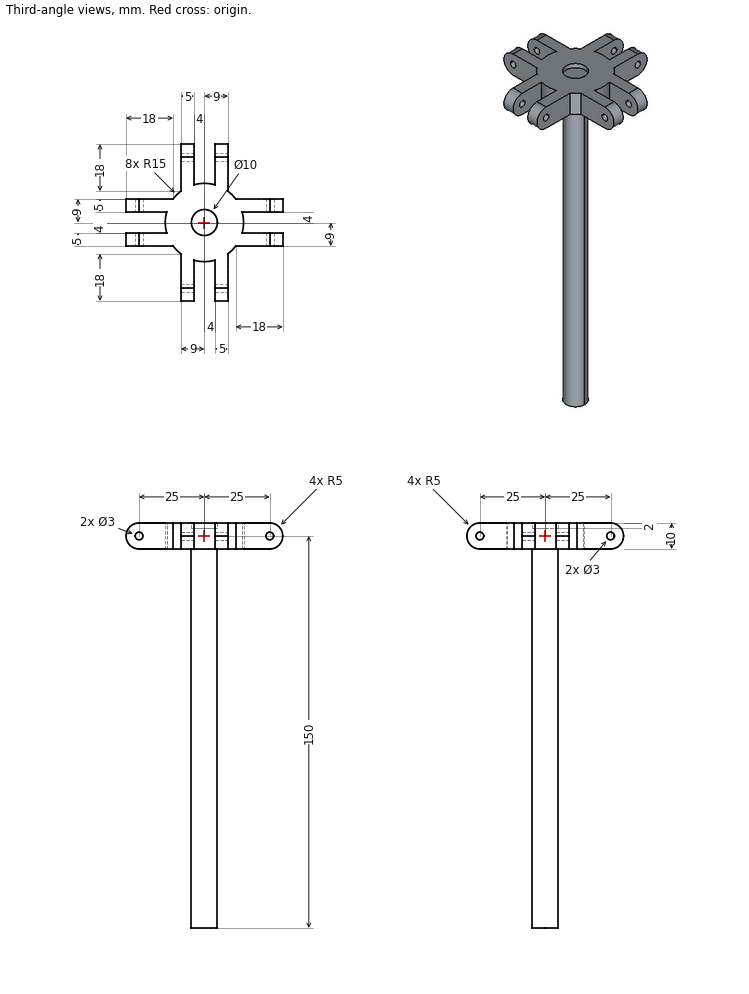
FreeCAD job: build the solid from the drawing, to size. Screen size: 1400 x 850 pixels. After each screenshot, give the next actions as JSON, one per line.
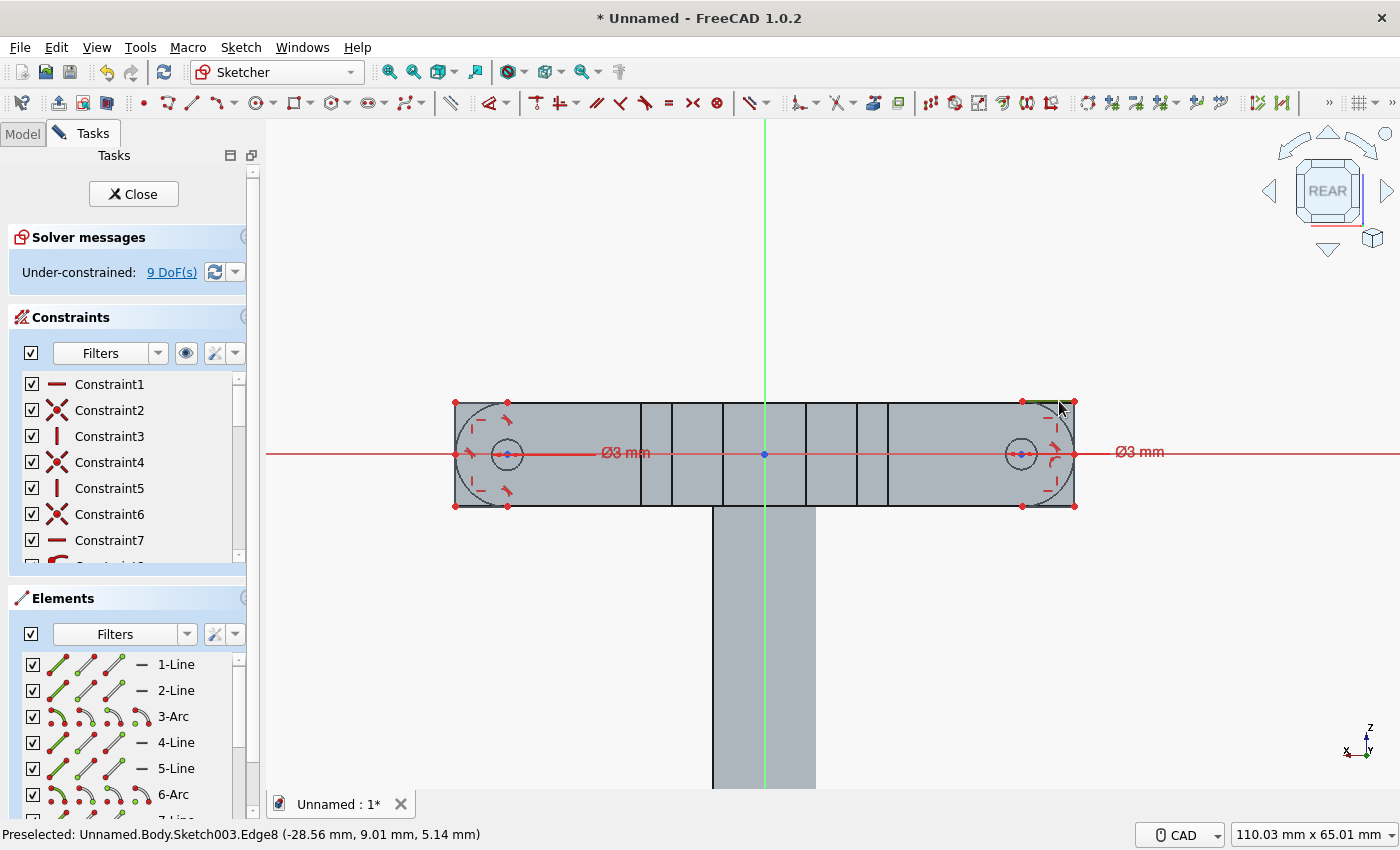
{"action": "left_click", "coordinate": [1059, 417]}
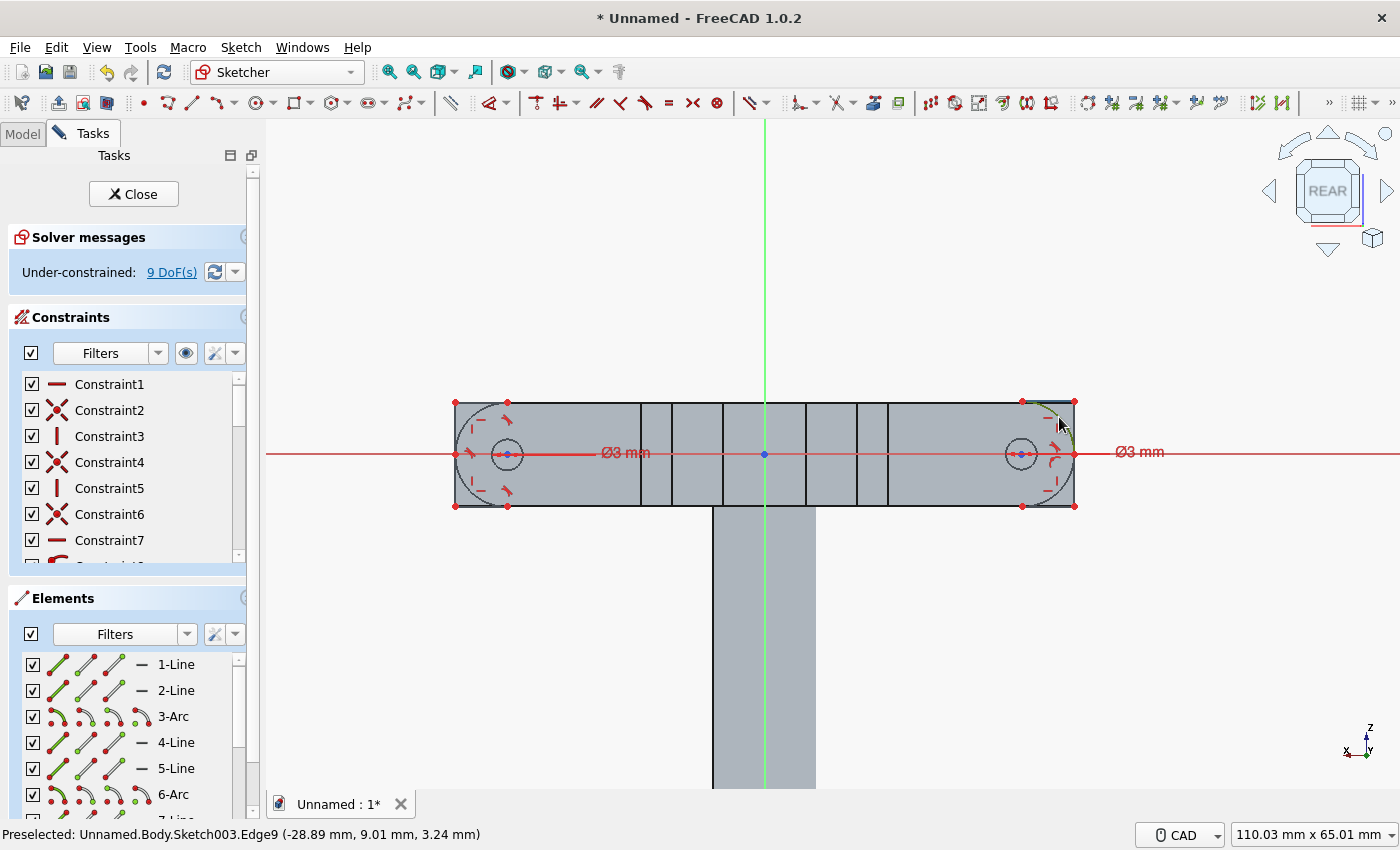
{"action": "key", "text": "t"}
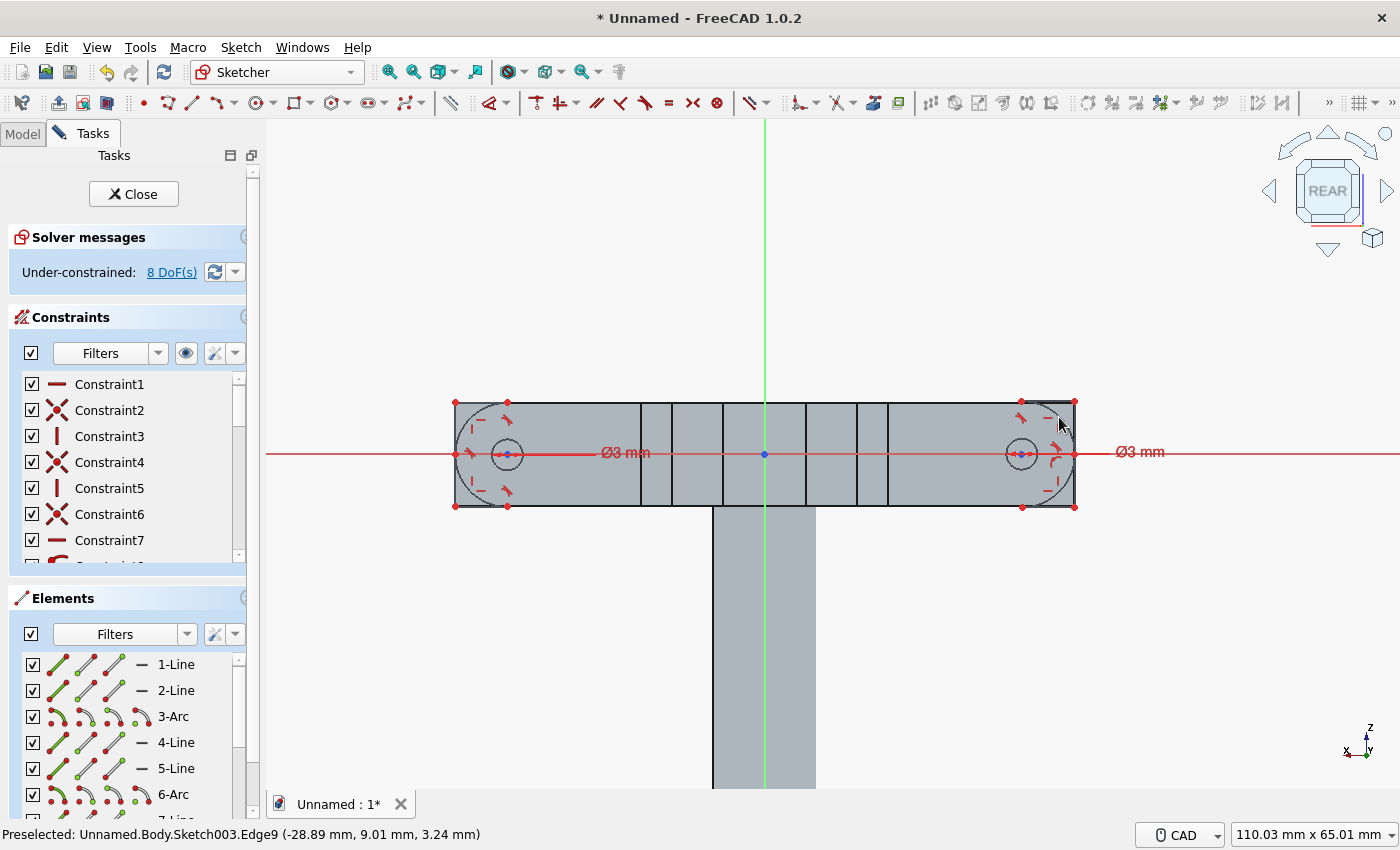
{"action": "left_click", "coordinate": [1059, 507]}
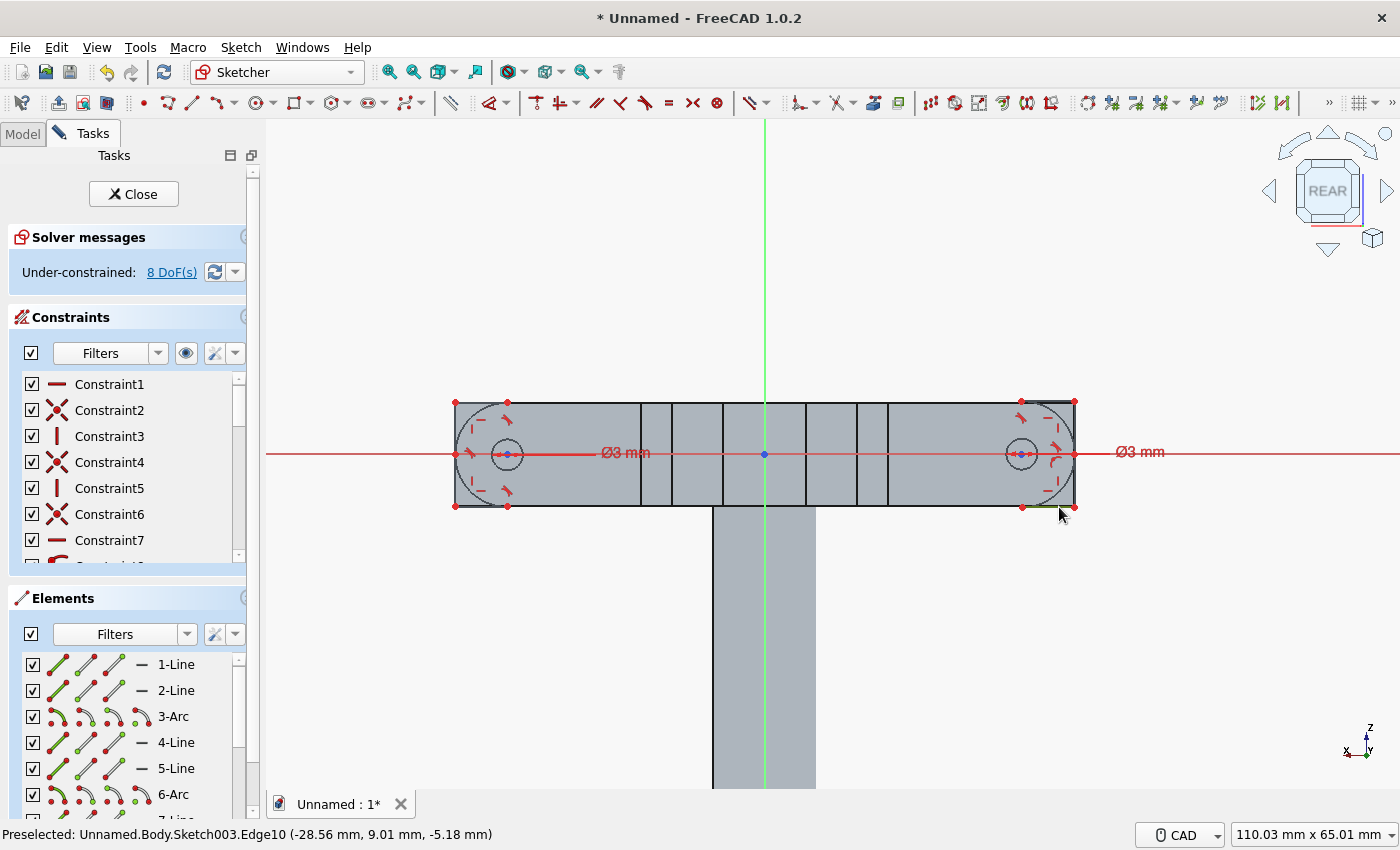
{"action": "left_click", "coordinate": [1059, 492]}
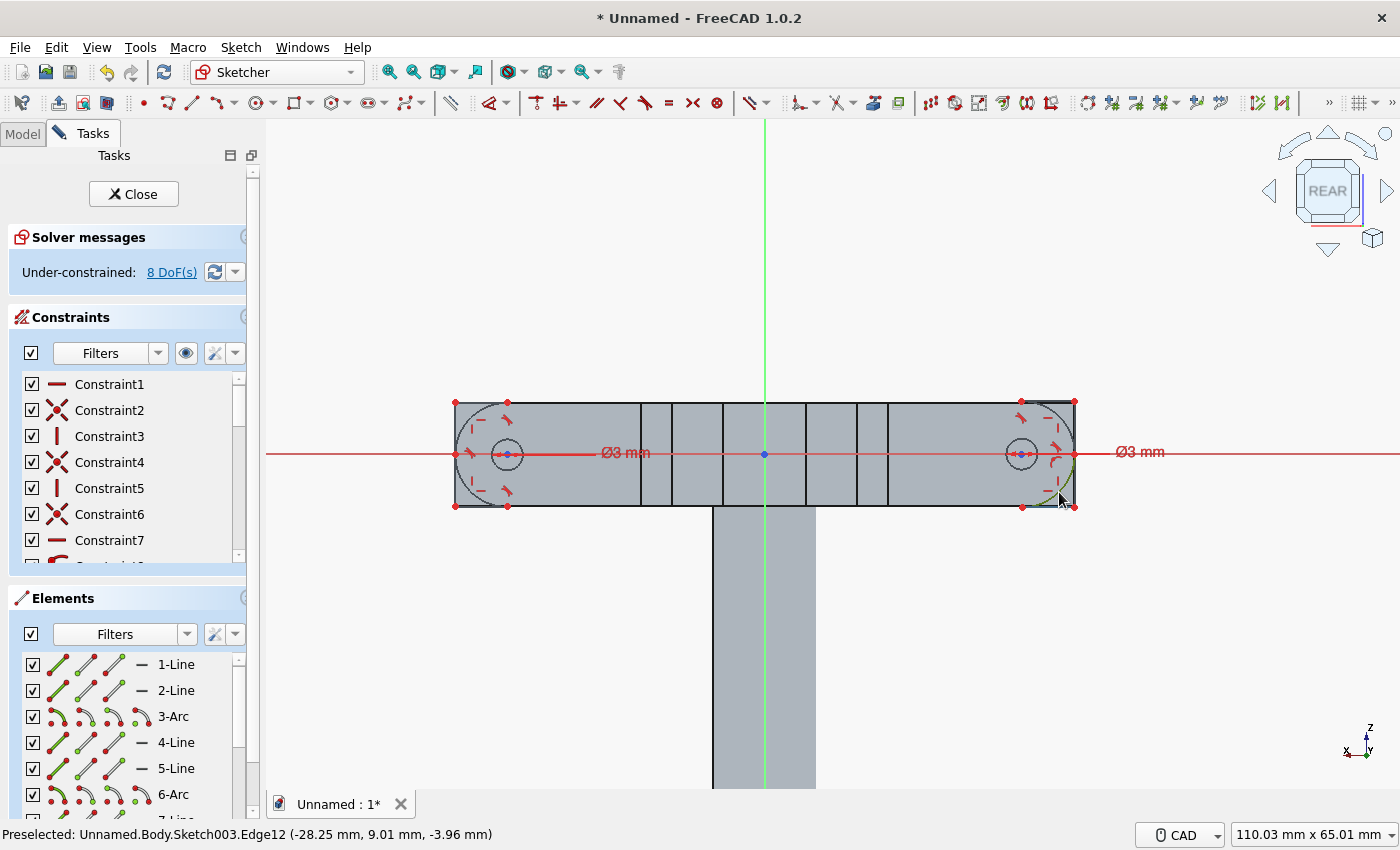
{"action": "key", "text": "t"}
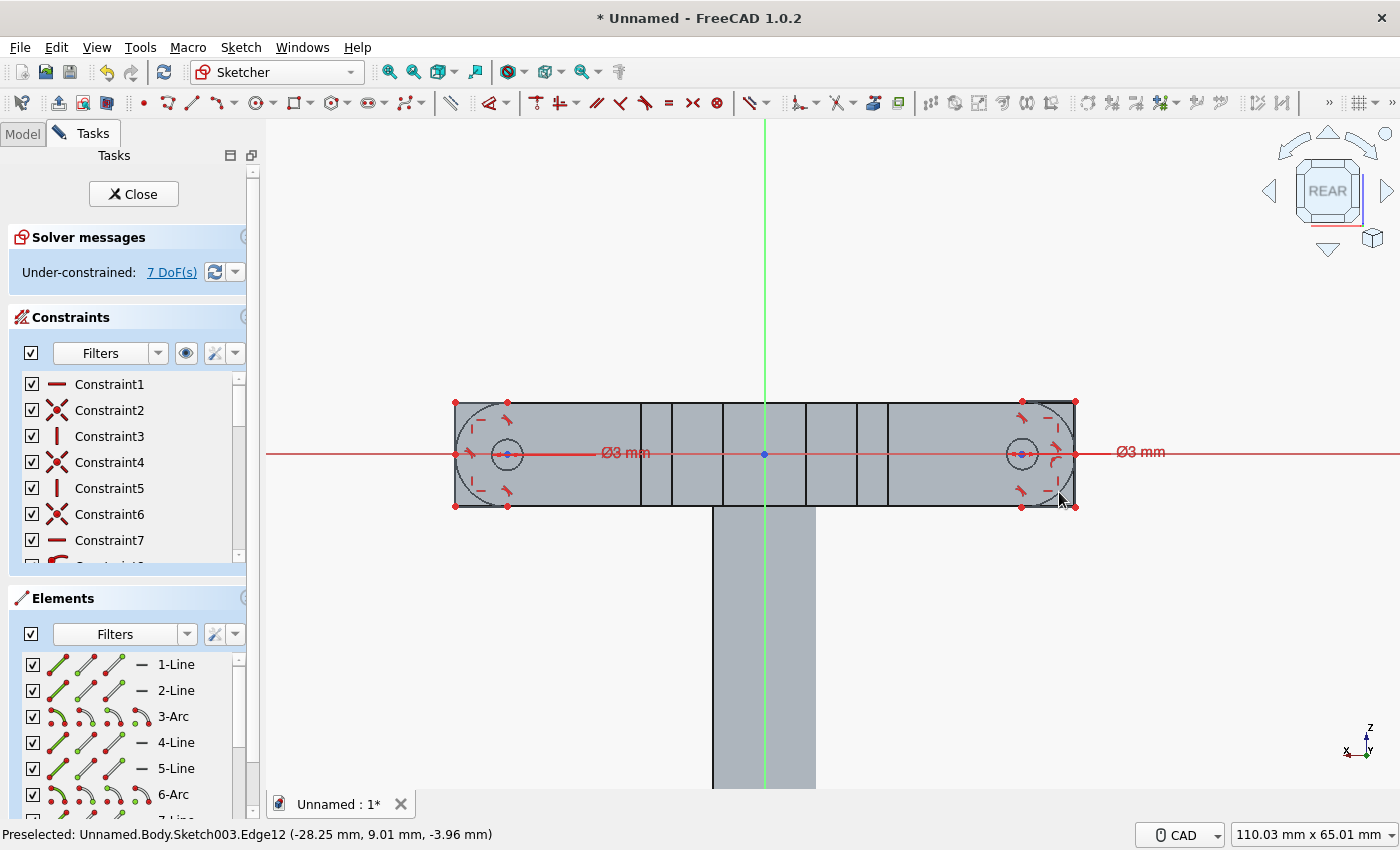
{"action": "left_click", "coordinate": [471, 418]}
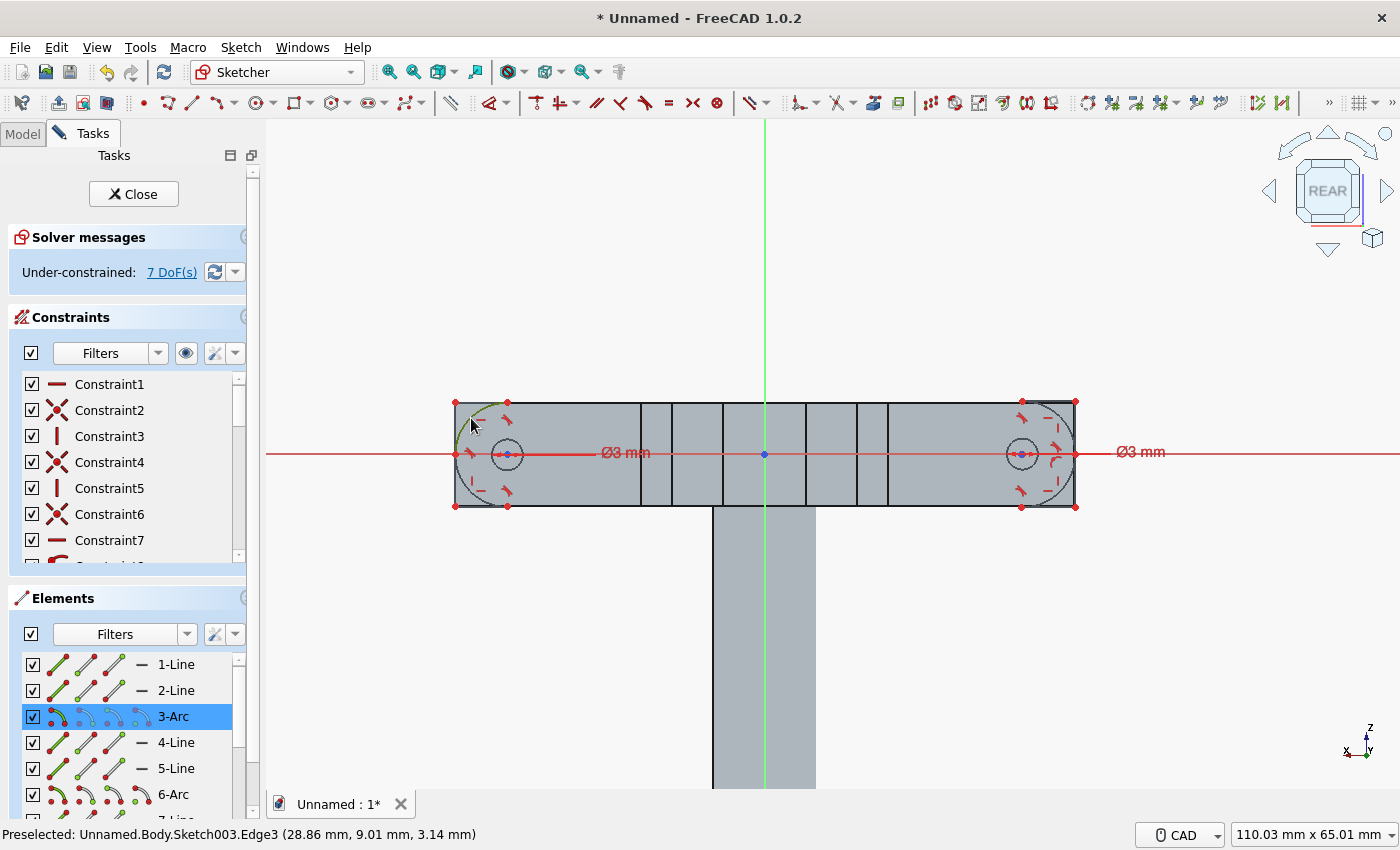
{"action": "left_click", "coordinate": [471, 492]}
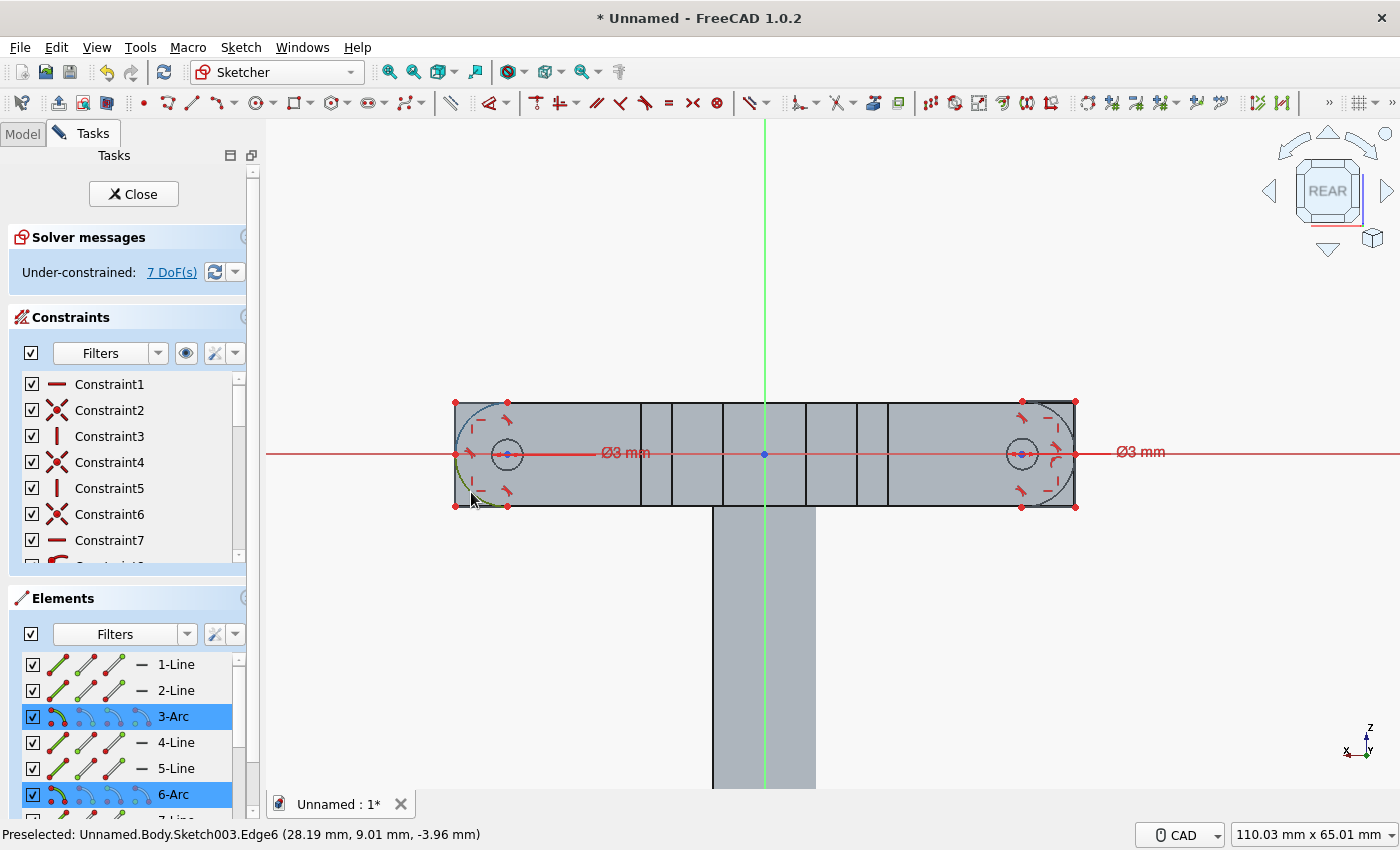
{"action": "left_click", "coordinate": [1060, 417]}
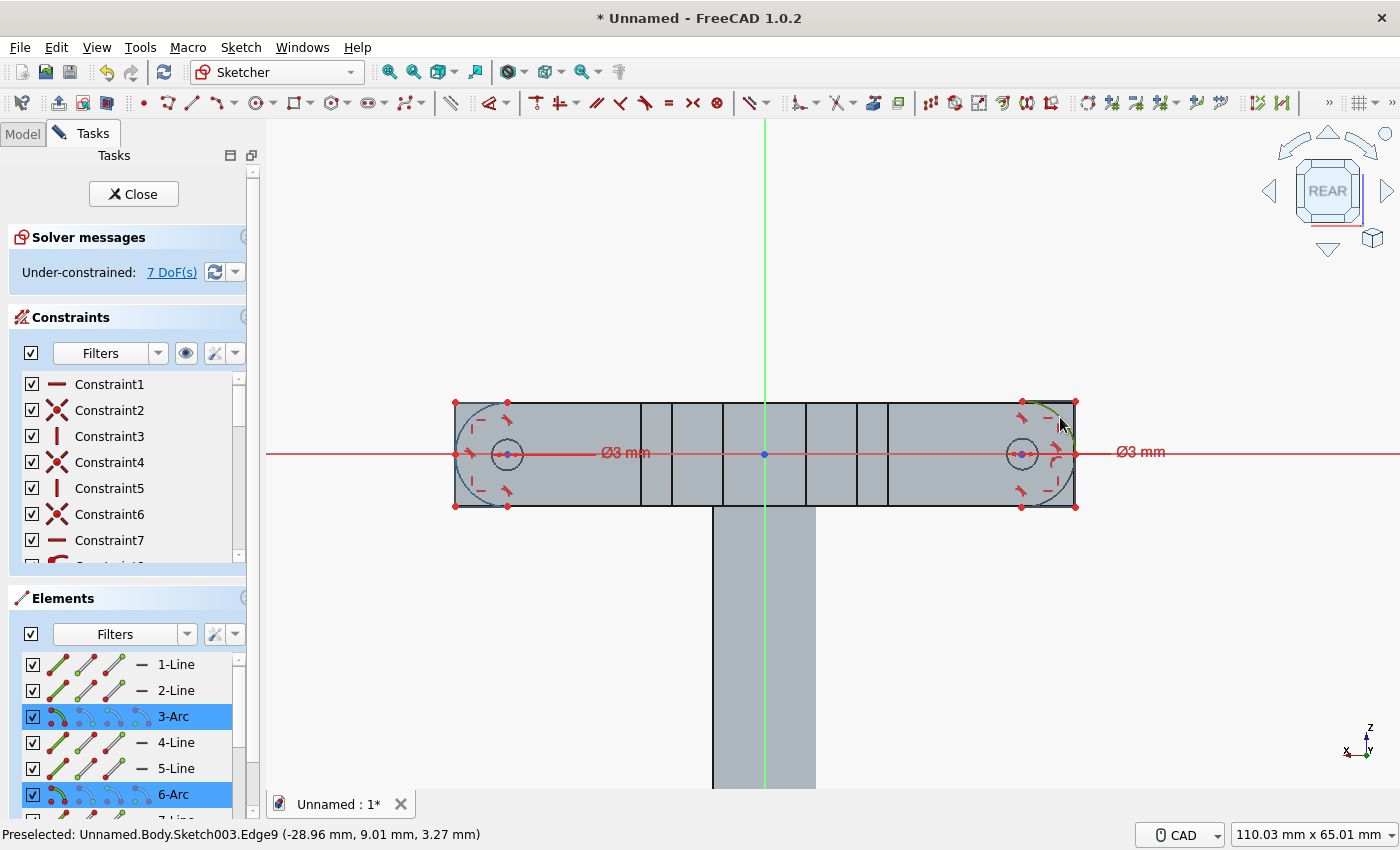
{"action": "left_click", "coordinate": [1060, 492]}